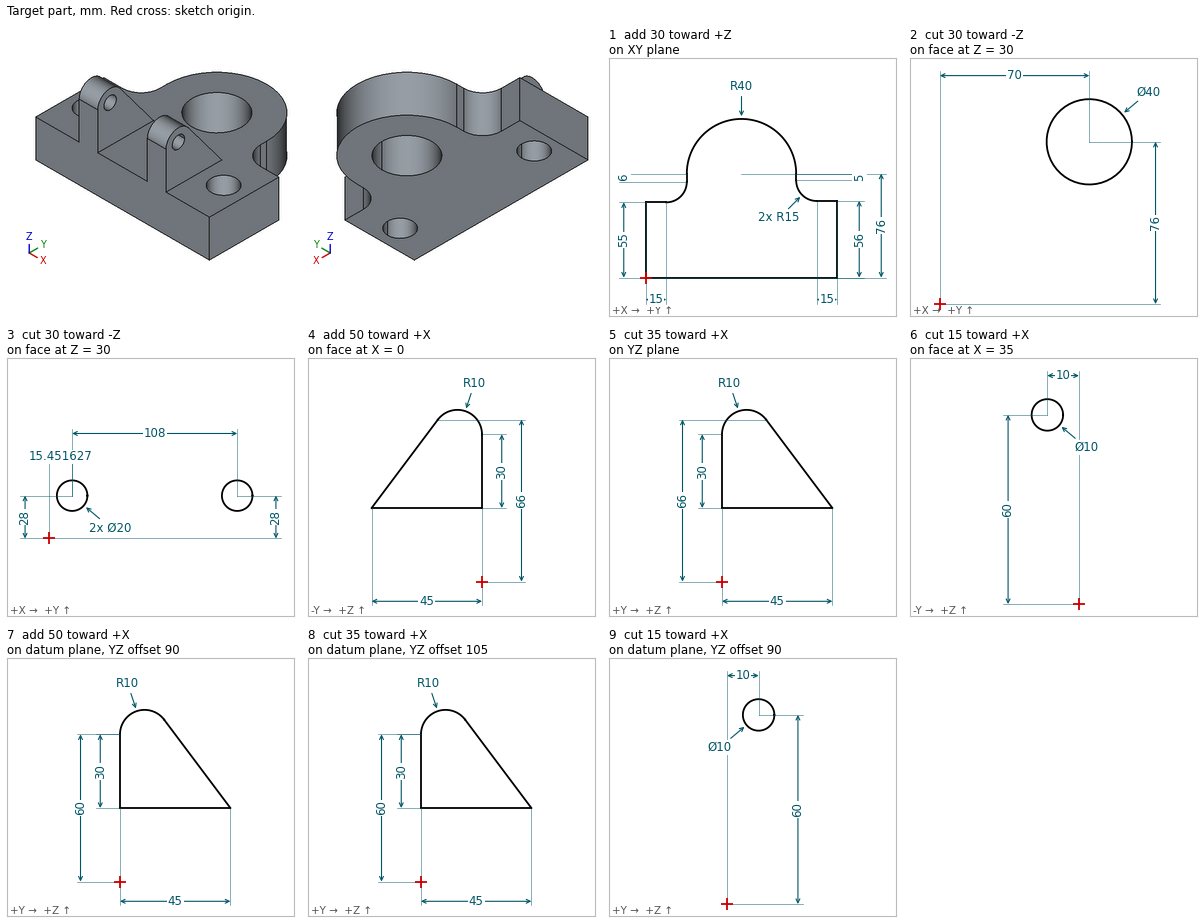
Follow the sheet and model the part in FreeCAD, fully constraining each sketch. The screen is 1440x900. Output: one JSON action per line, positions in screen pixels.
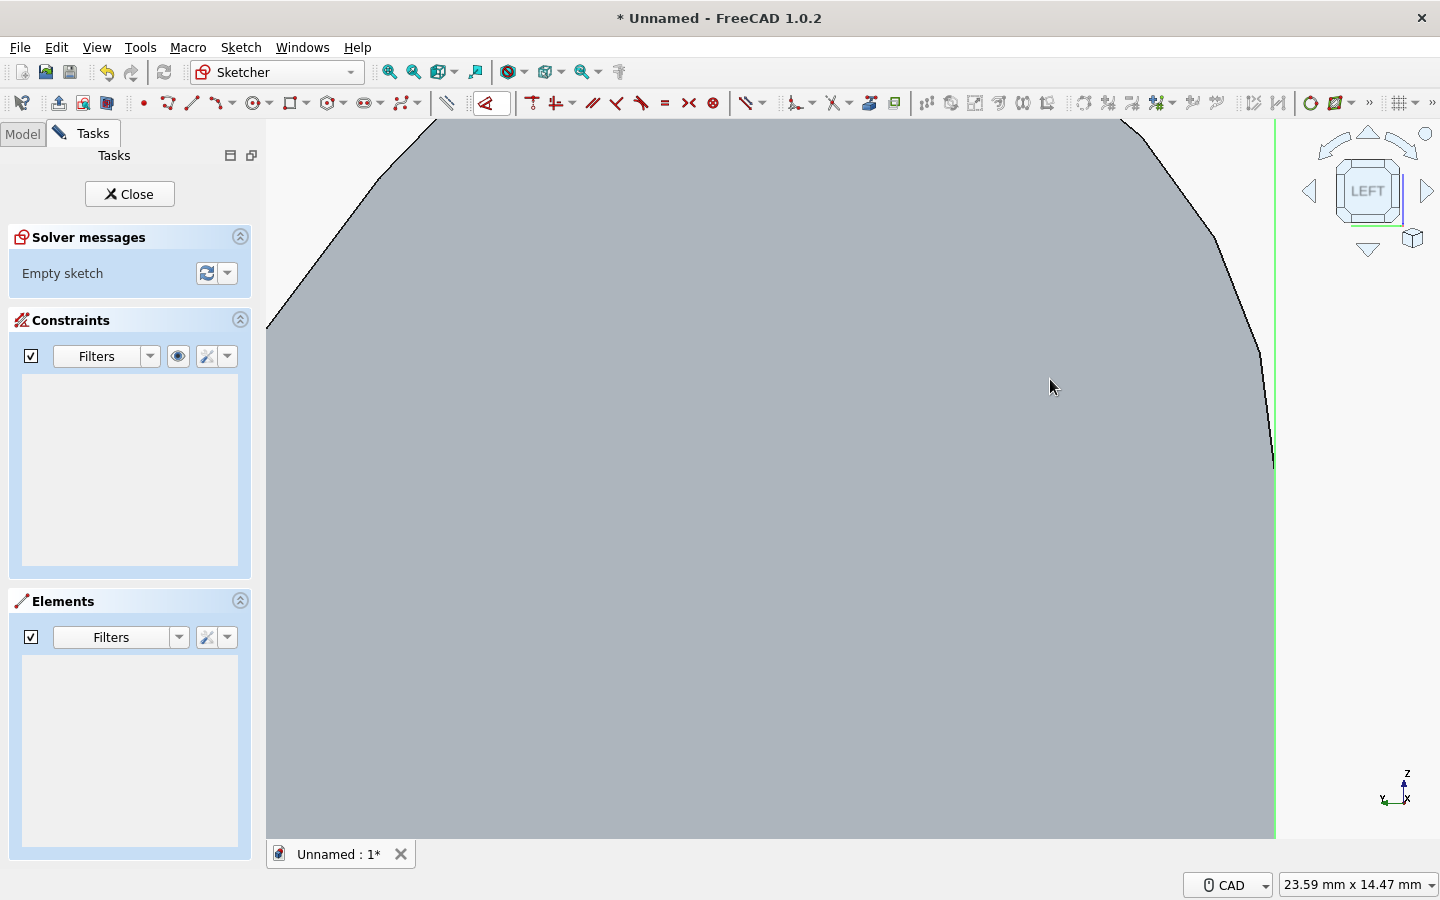
{"action": "key", "text": "g c"}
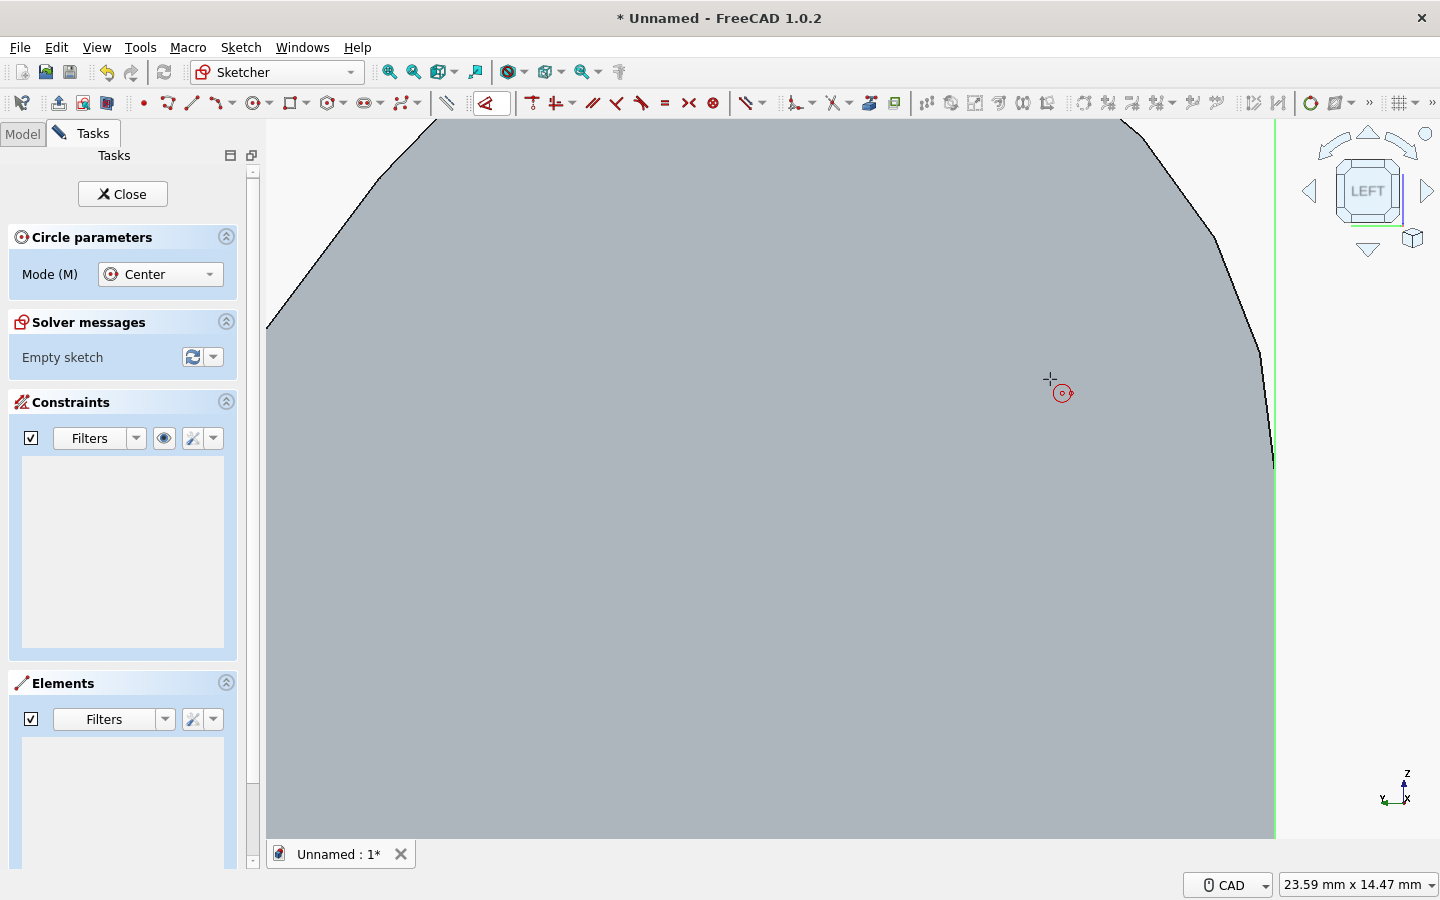
{"action": "left_click", "coordinate": [778, 476]}
{"action": "mouse_move", "coordinate": [954, 300]}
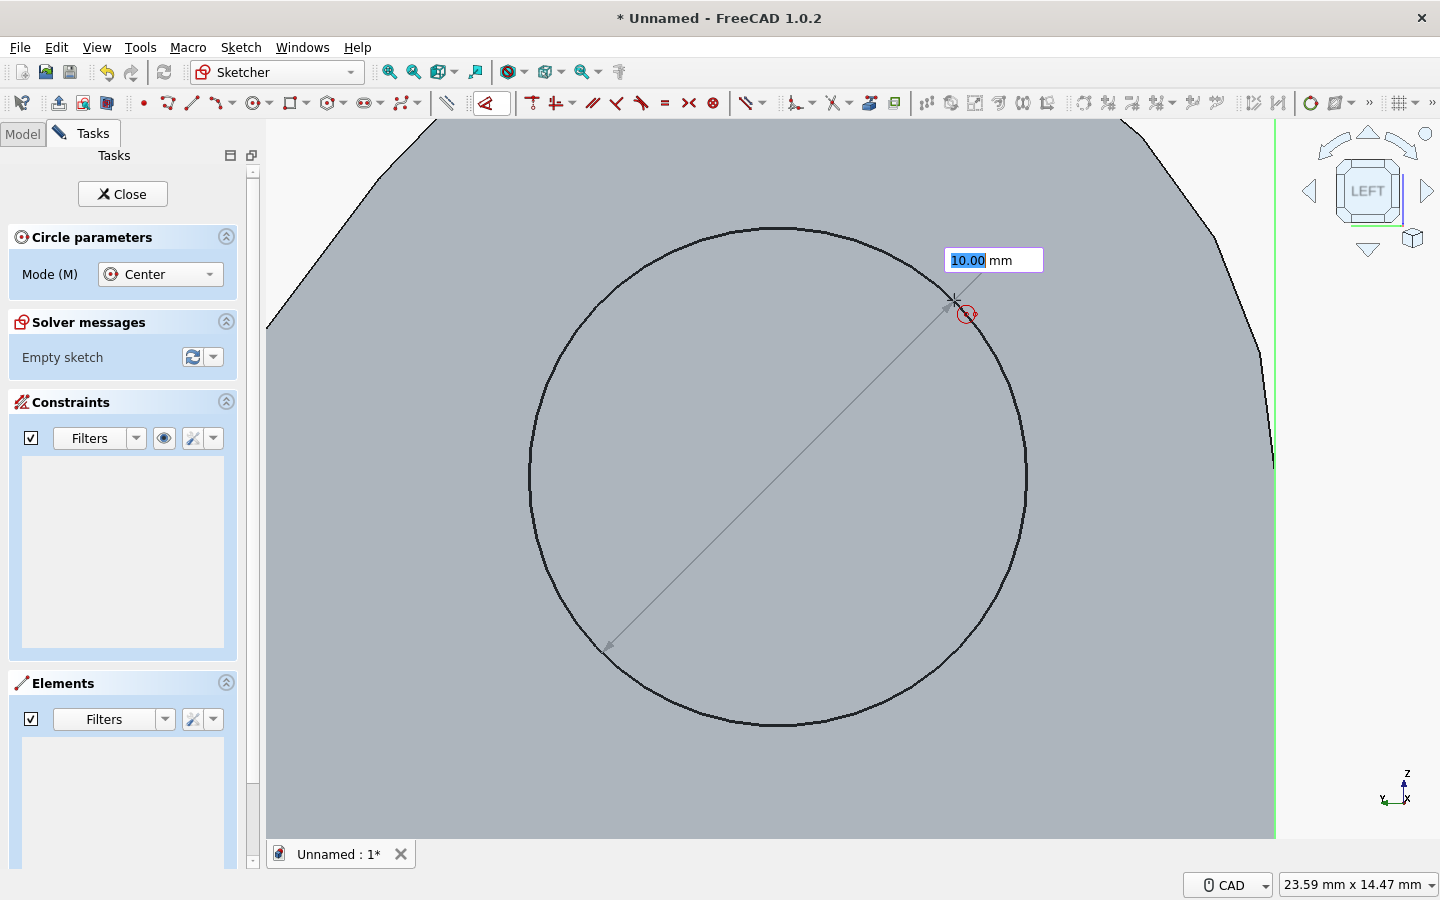
{"action": "type", "text": "10"}
{"action": "key", "text": "Return"}
{"action": "key", "text": "Escape"}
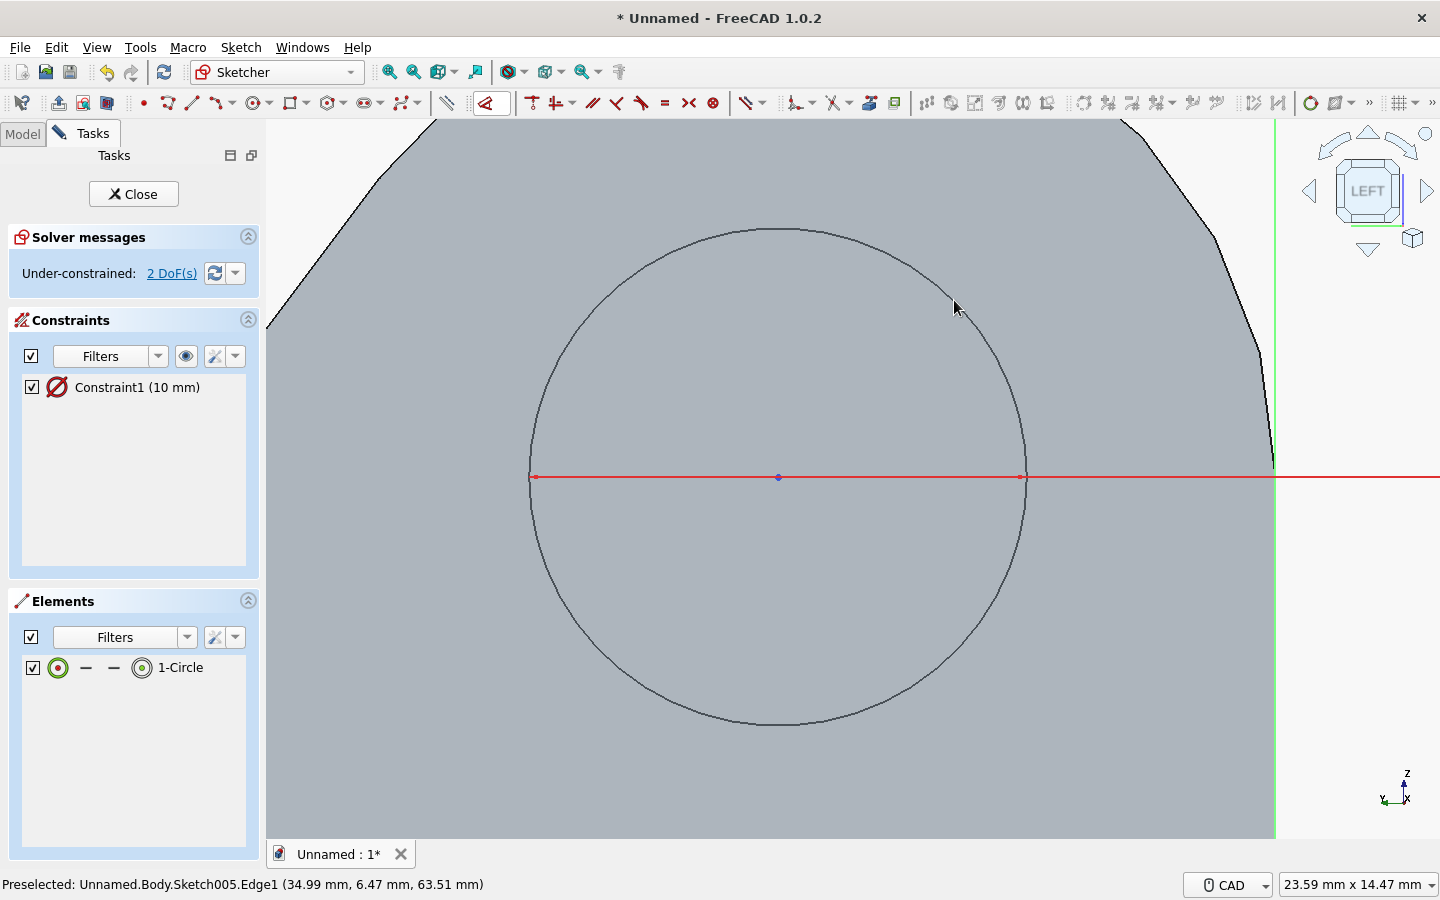
{"action": "left_click", "coordinate": [778, 477]}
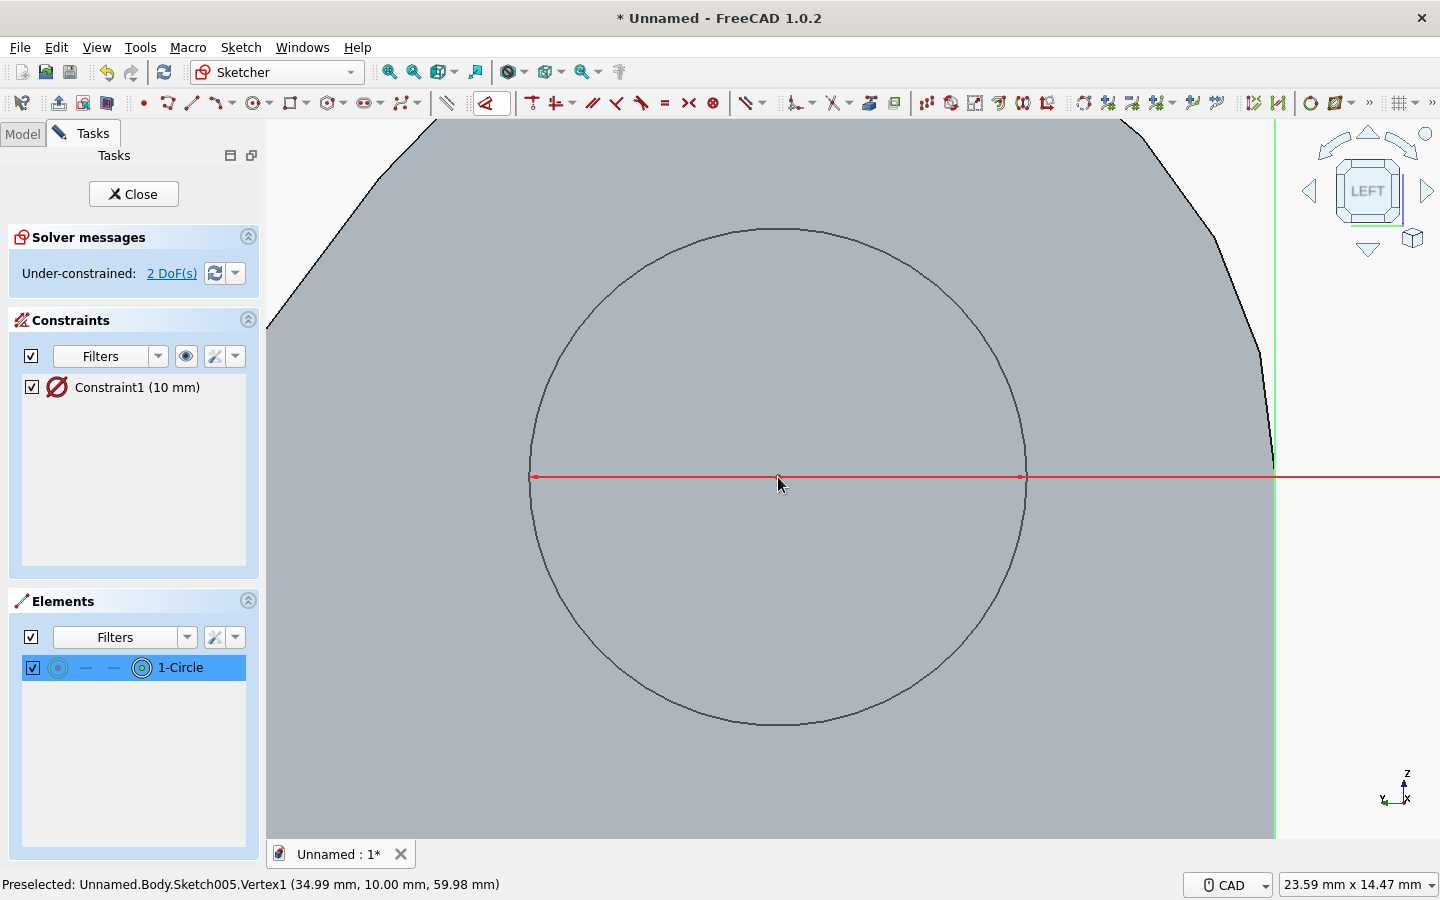
{"action": "key", "text": "l"}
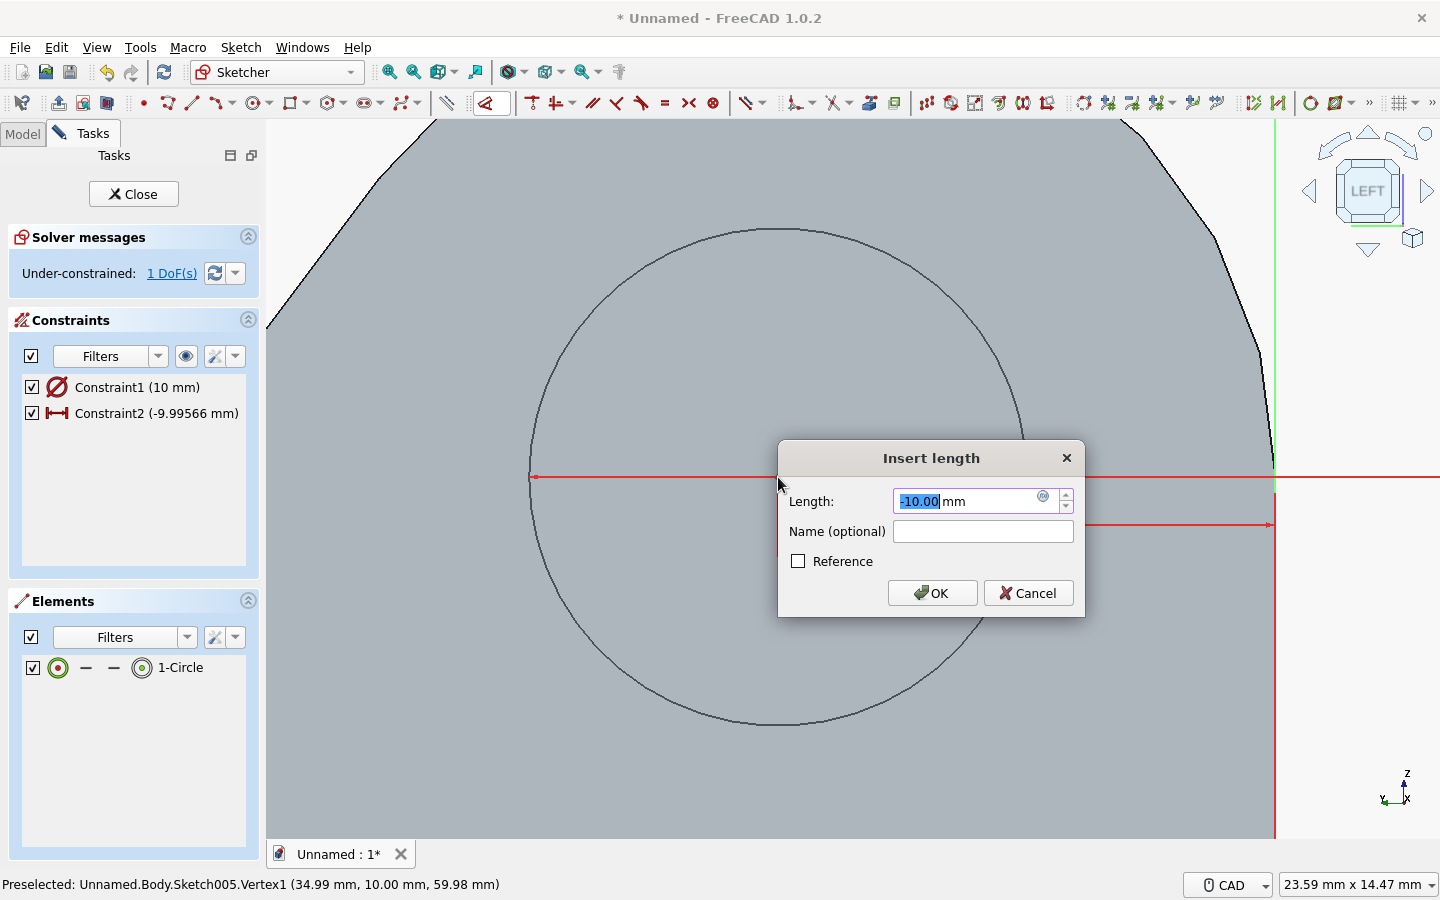
{"action": "type", "text": "-10"}
{"action": "key", "text": "Return"}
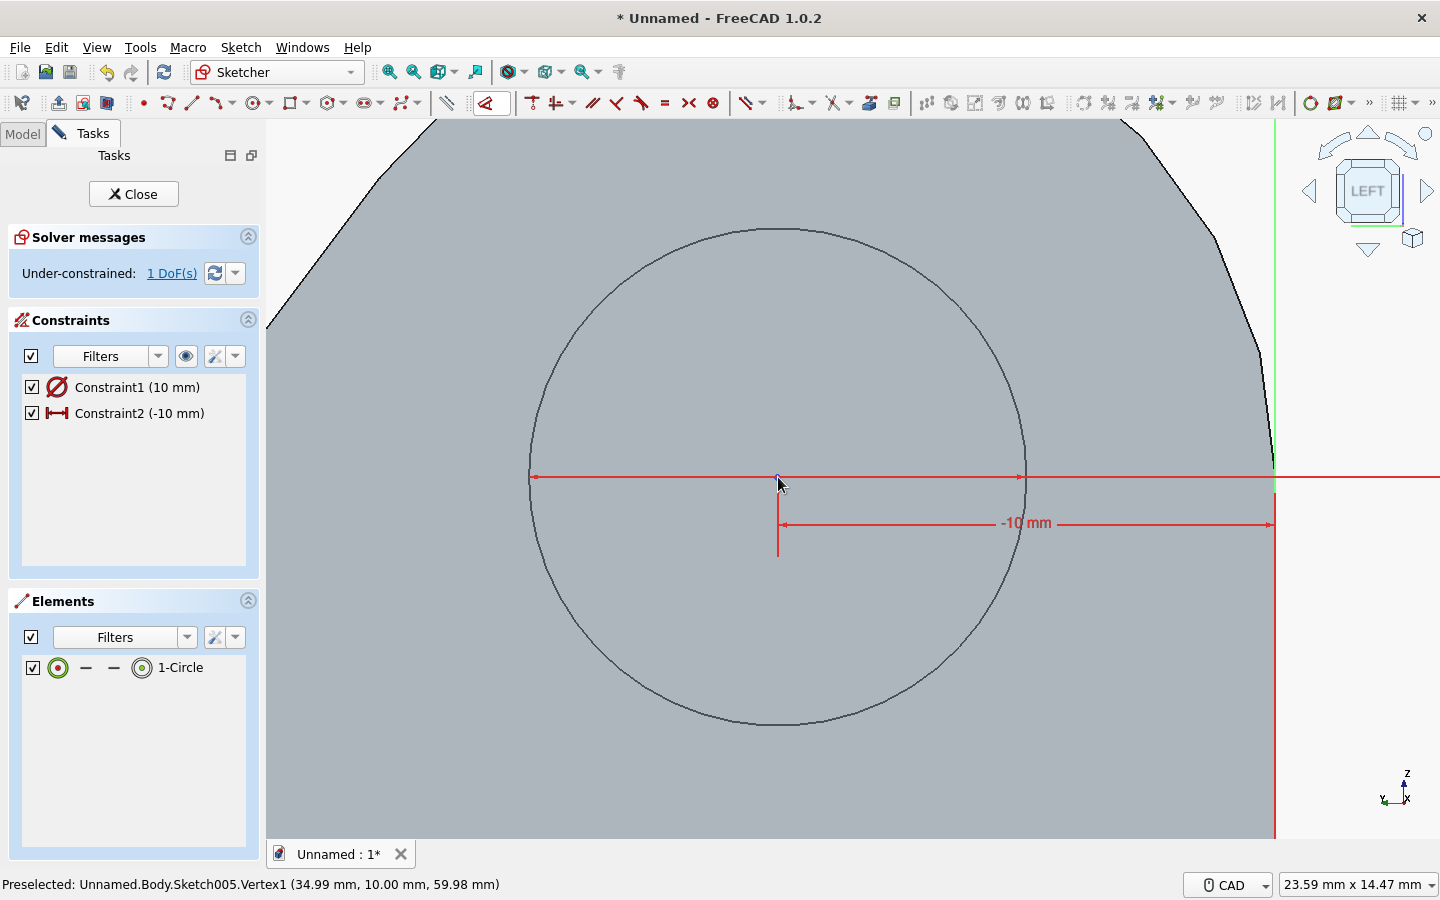
{"action": "left_click", "coordinate": [778, 477]}